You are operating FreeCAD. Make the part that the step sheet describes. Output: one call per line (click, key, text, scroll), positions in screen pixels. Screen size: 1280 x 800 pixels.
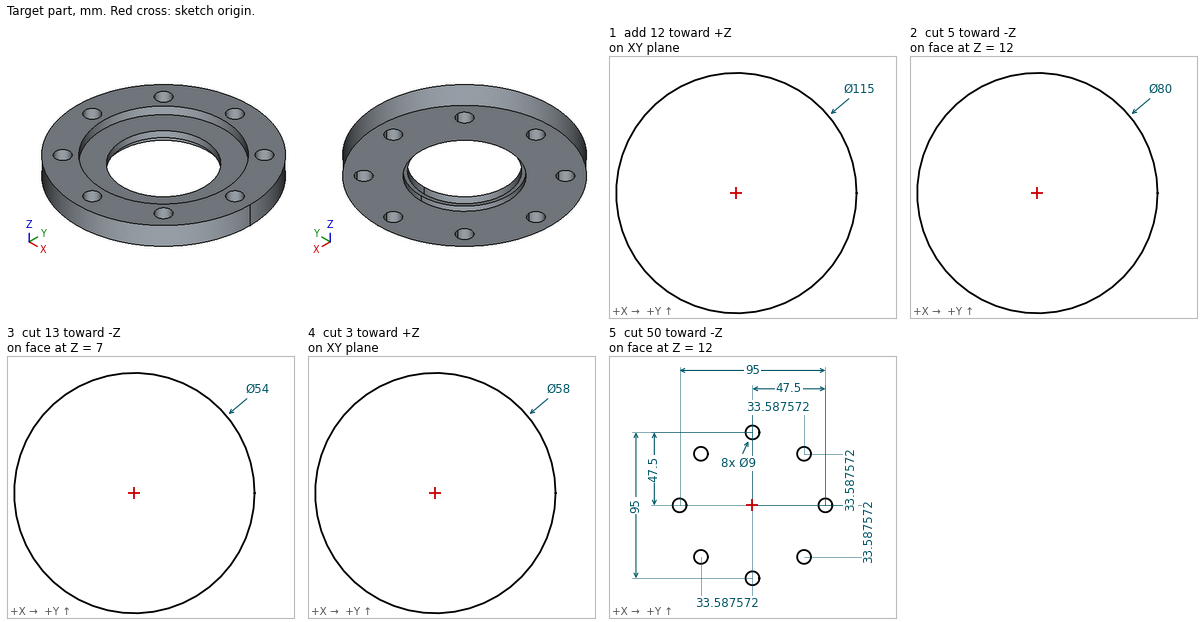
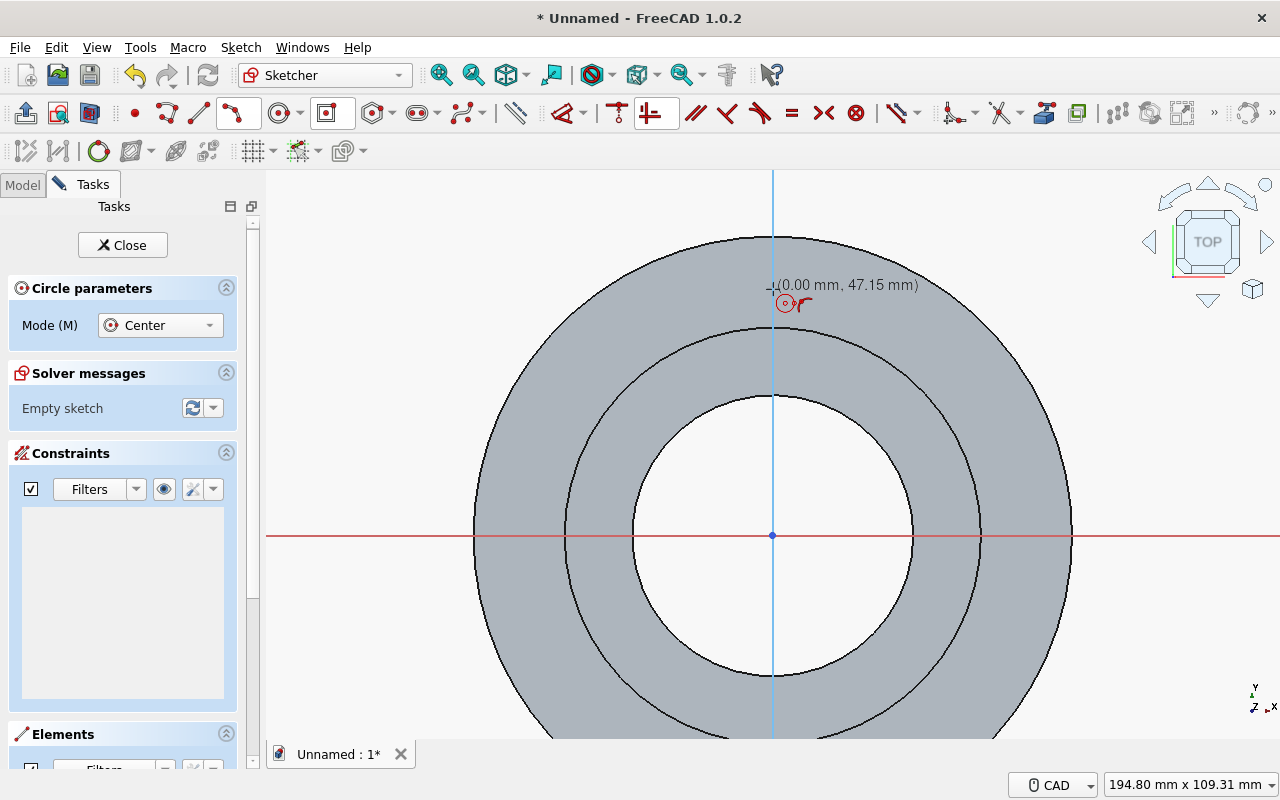
click(773, 289)
move(789, 272)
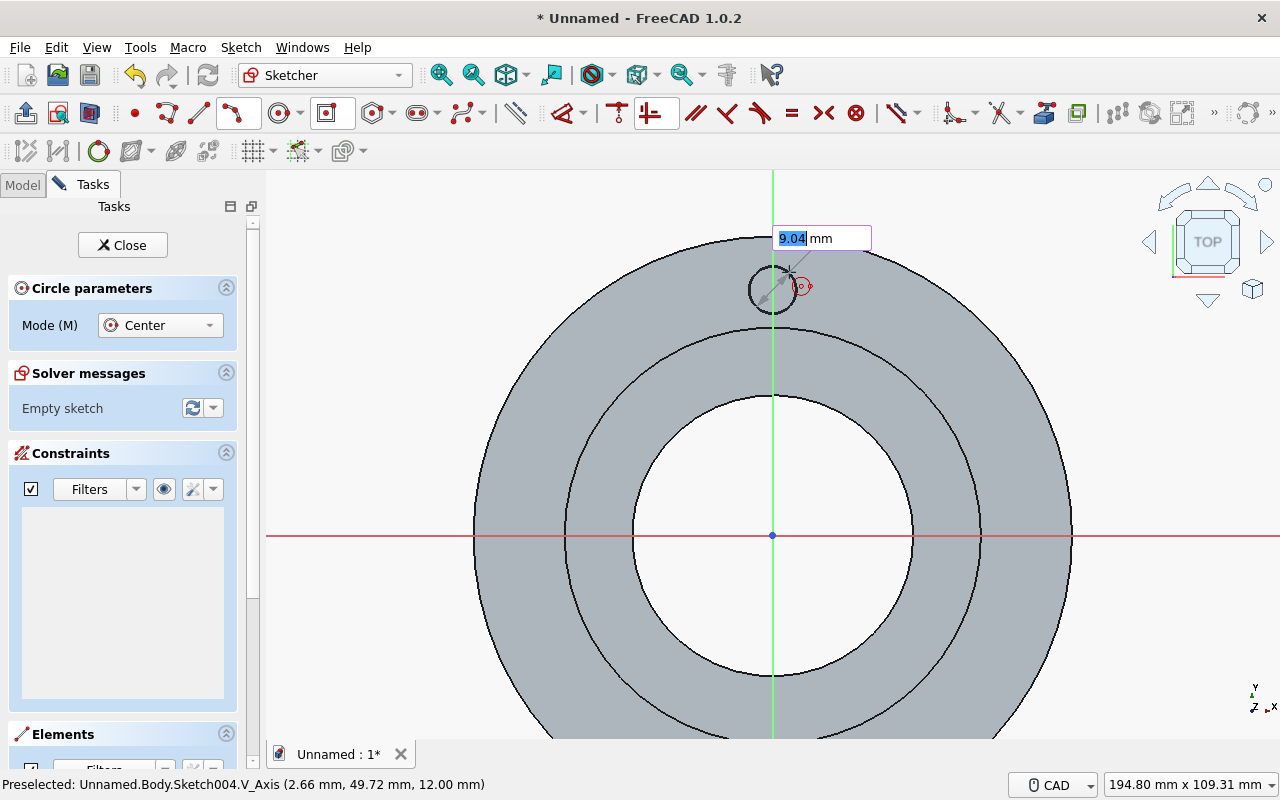
text(9)
key(Return)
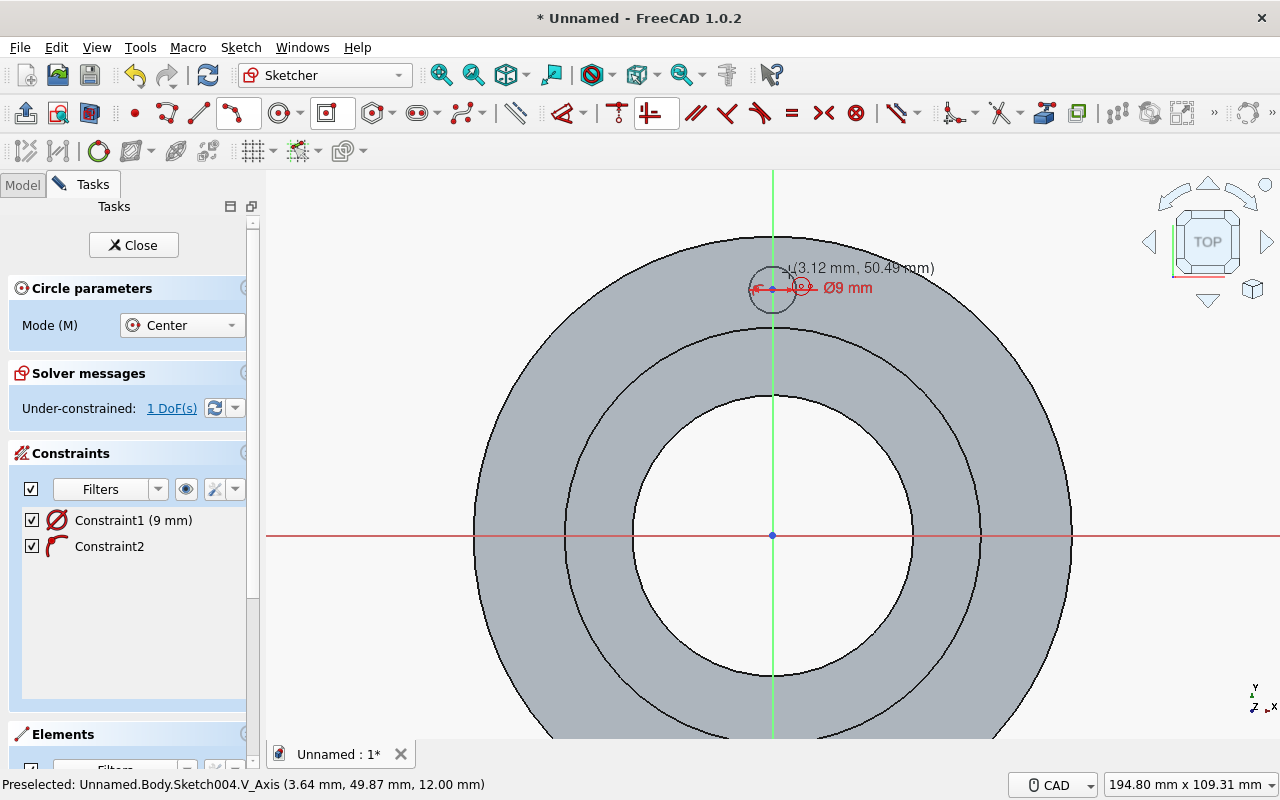
click(948, 361)
move(964, 344)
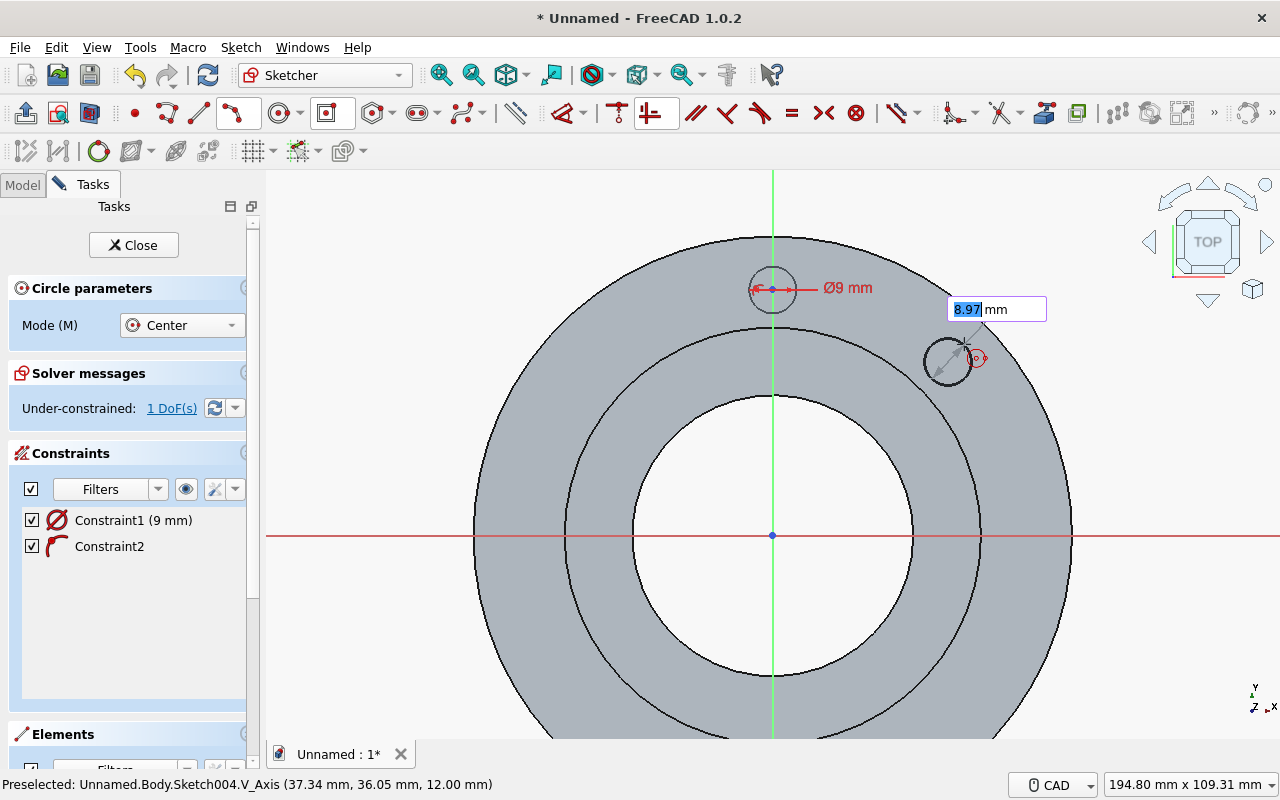
text(9)
key(Return)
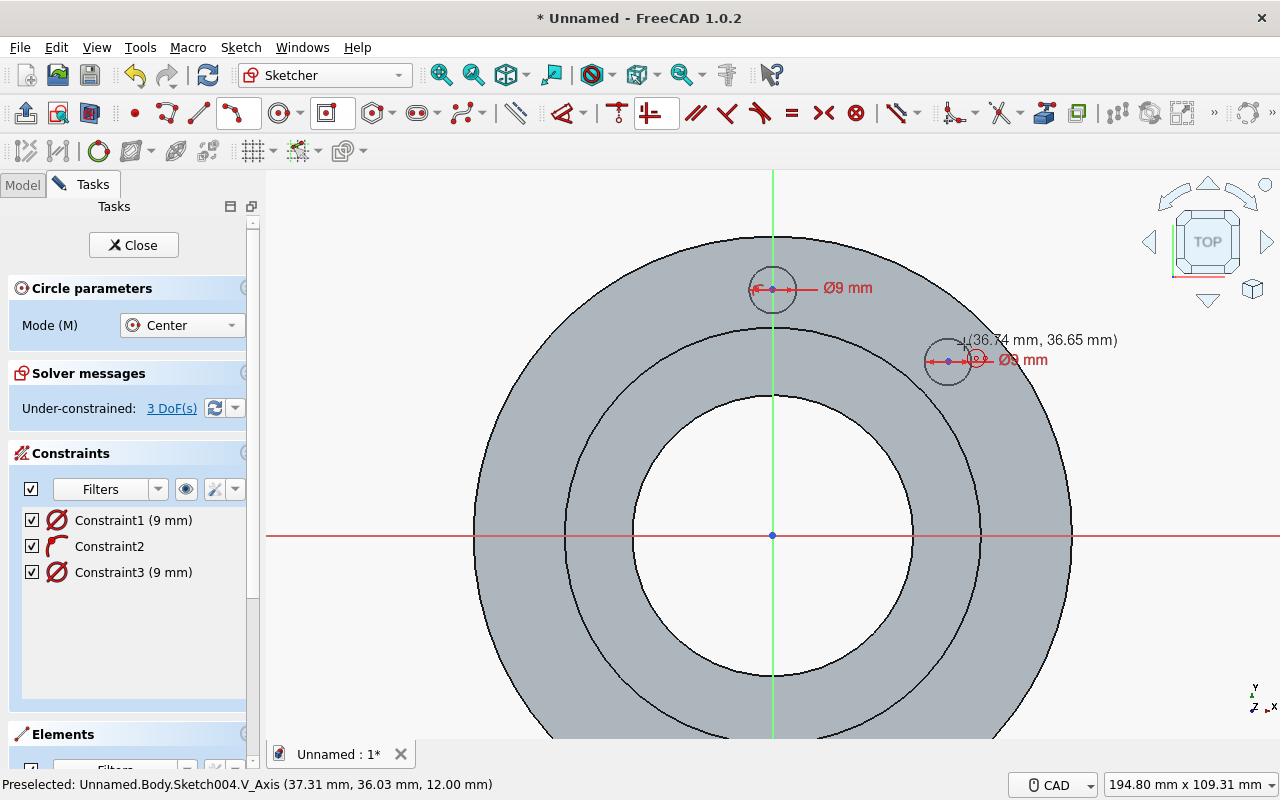
click(1020, 536)
move(1037, 519)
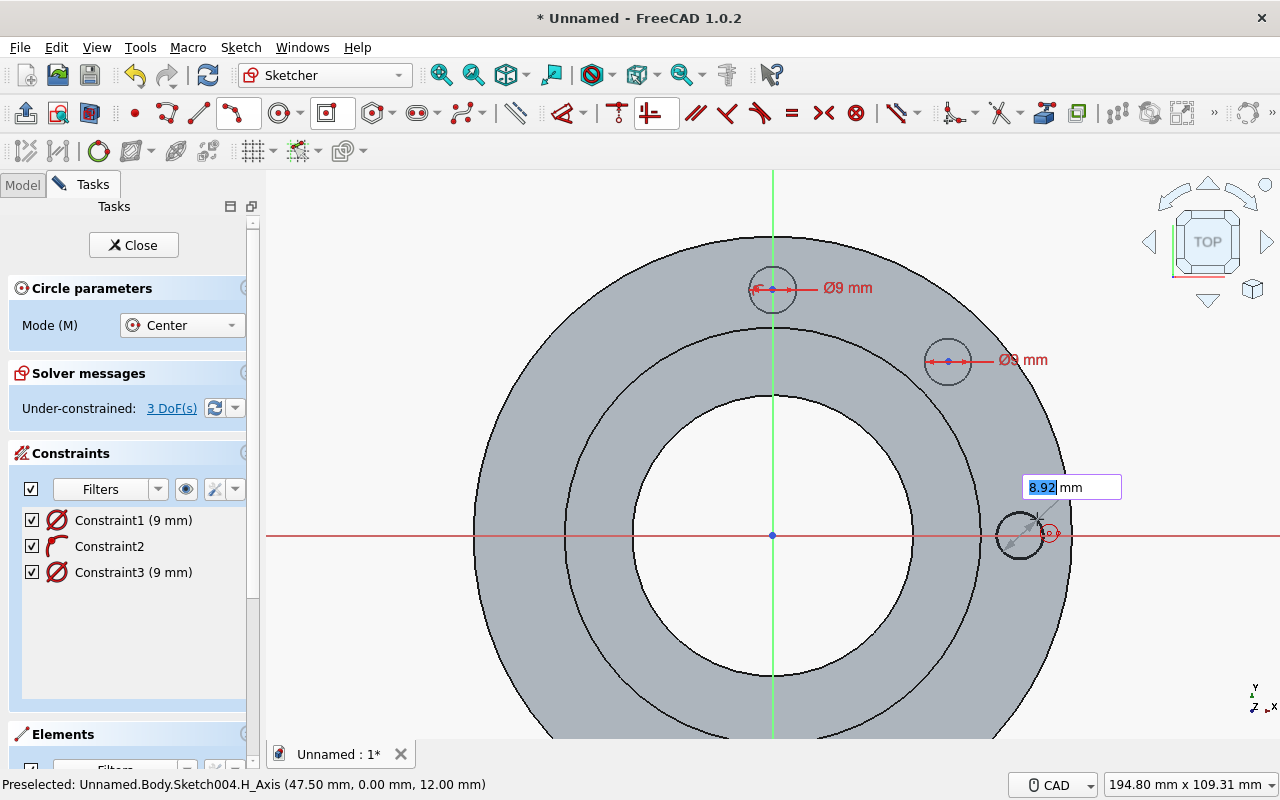
text(9)
key(Return)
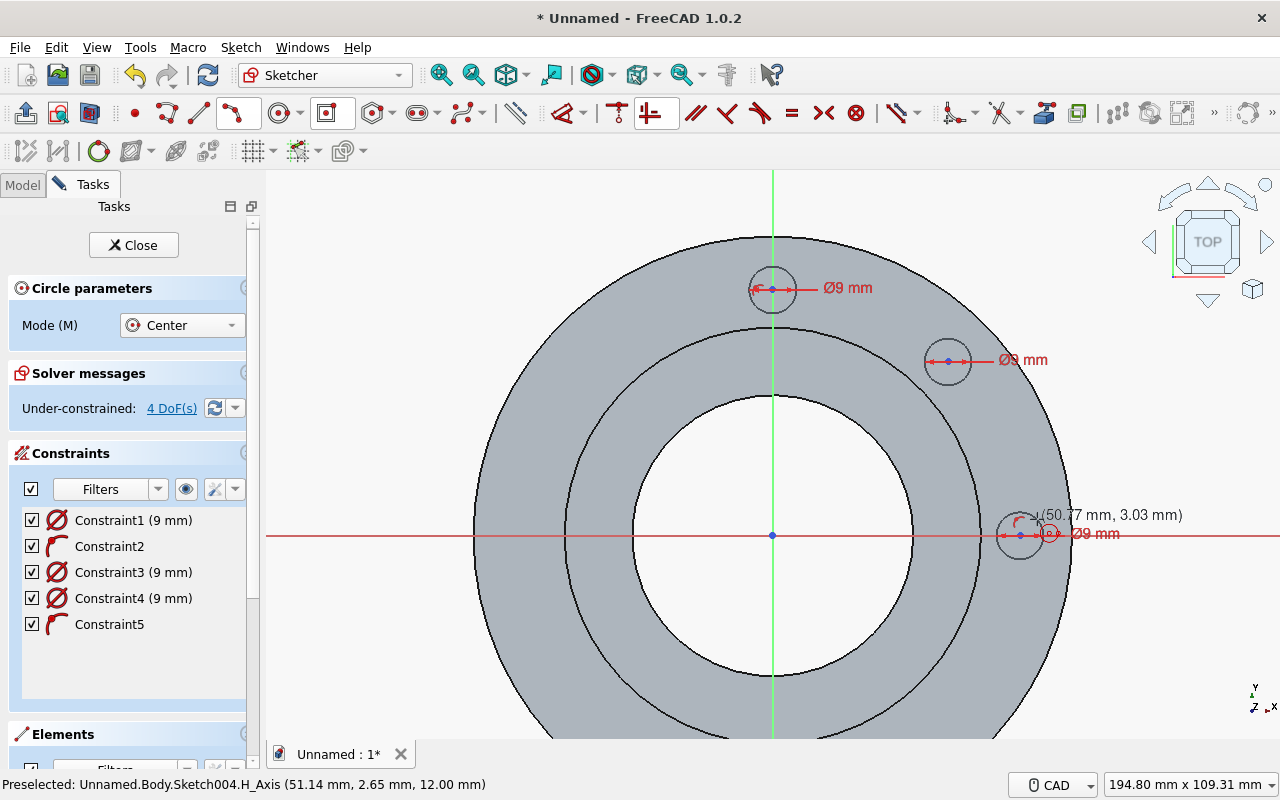
click(948, 711)
move(964, 694)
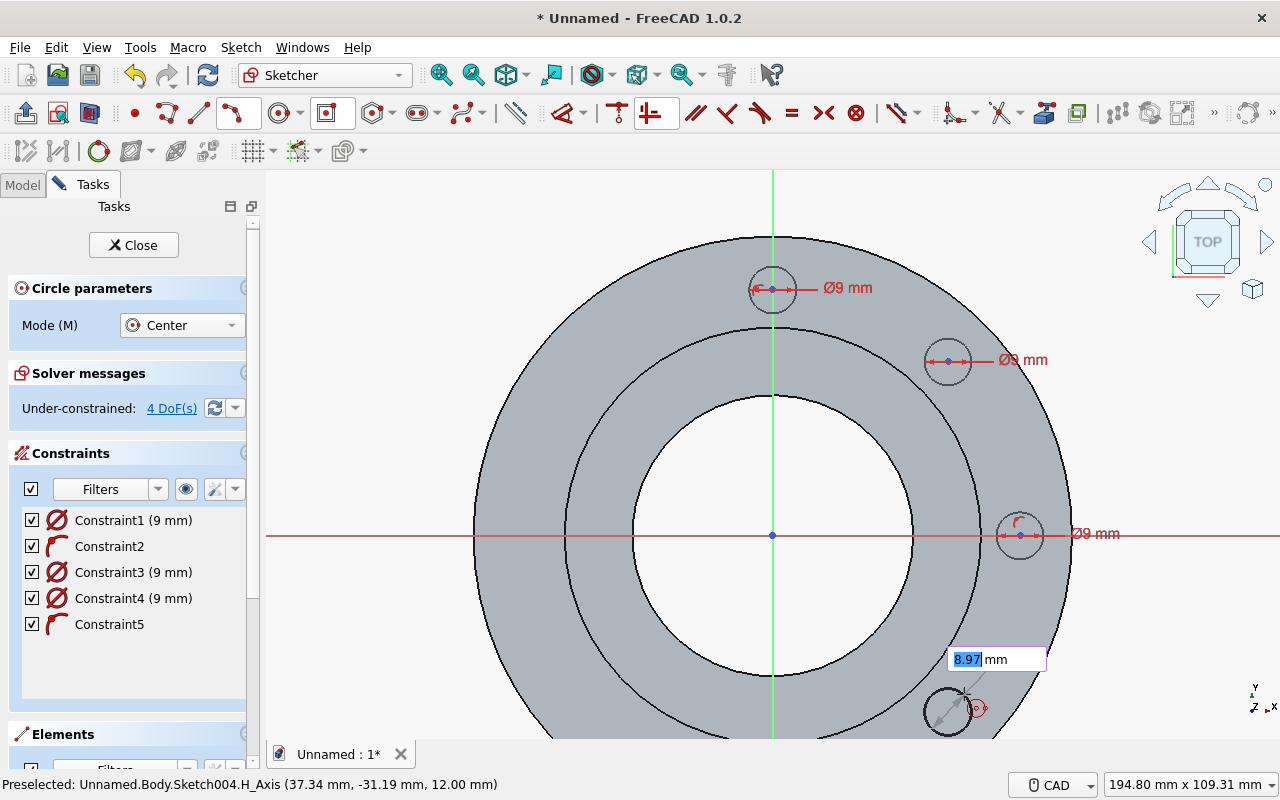
text(9)
key(Return)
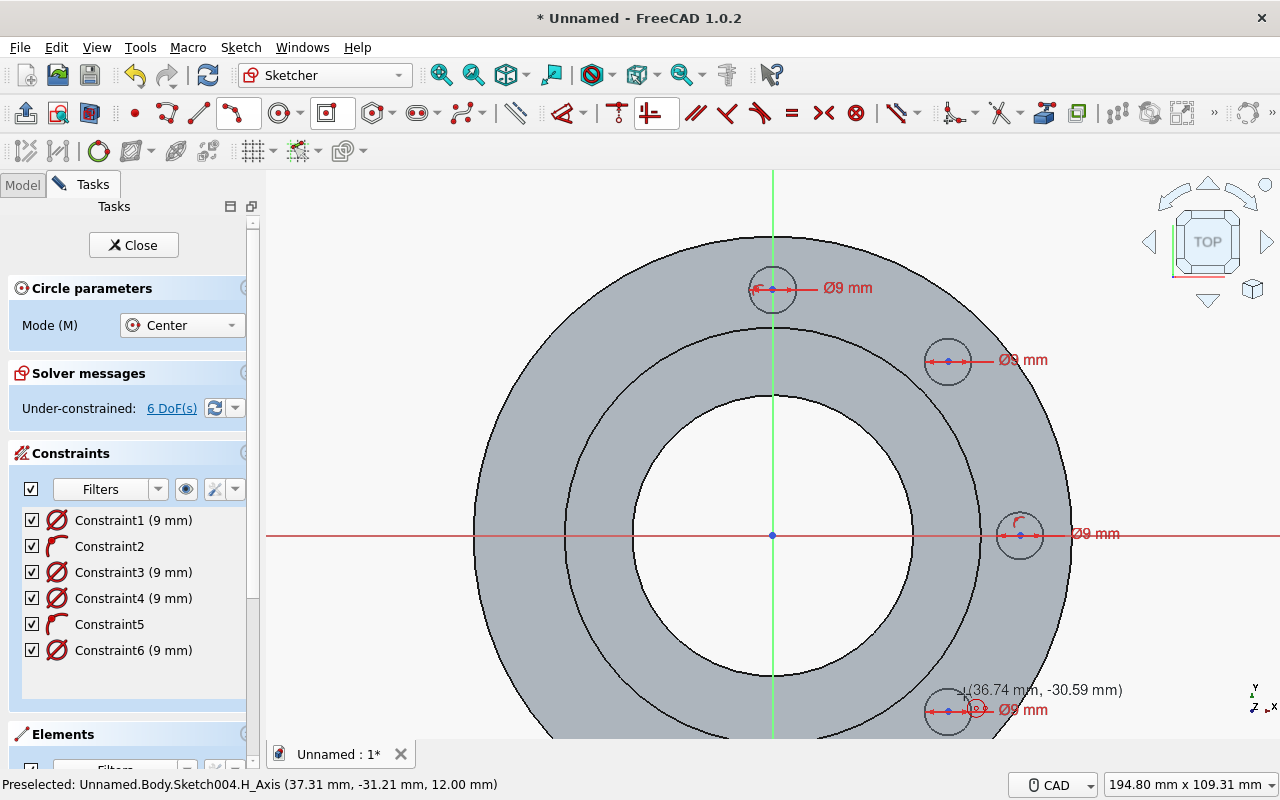
scroll(566, 289, down, 2)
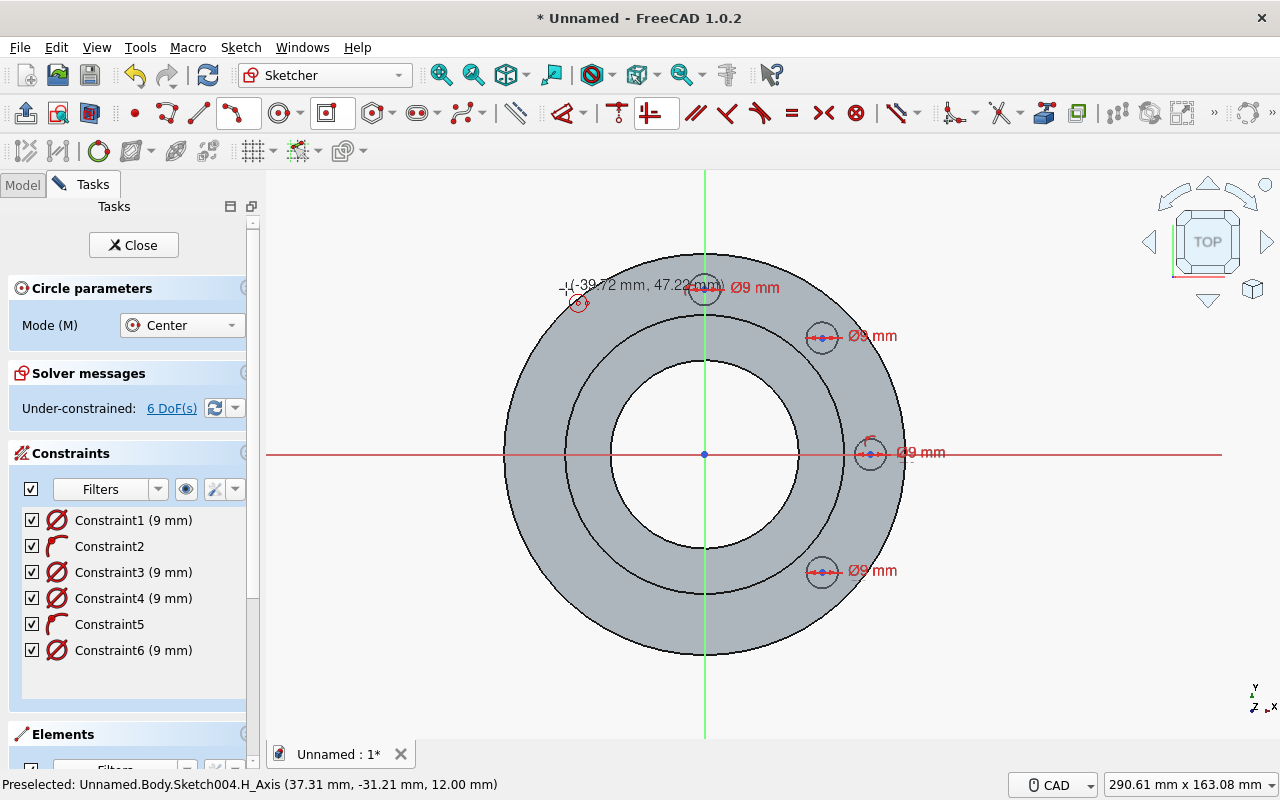
scroll(705, 620, up, 2)